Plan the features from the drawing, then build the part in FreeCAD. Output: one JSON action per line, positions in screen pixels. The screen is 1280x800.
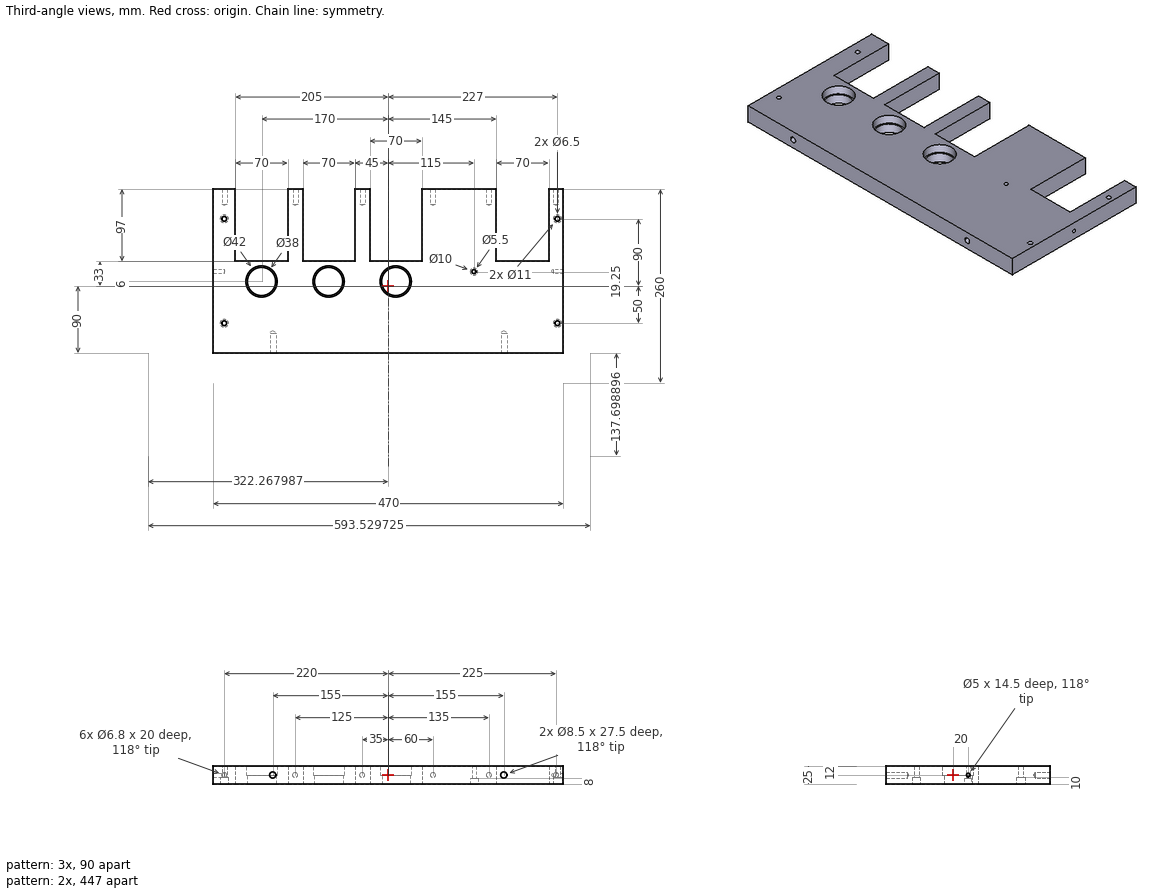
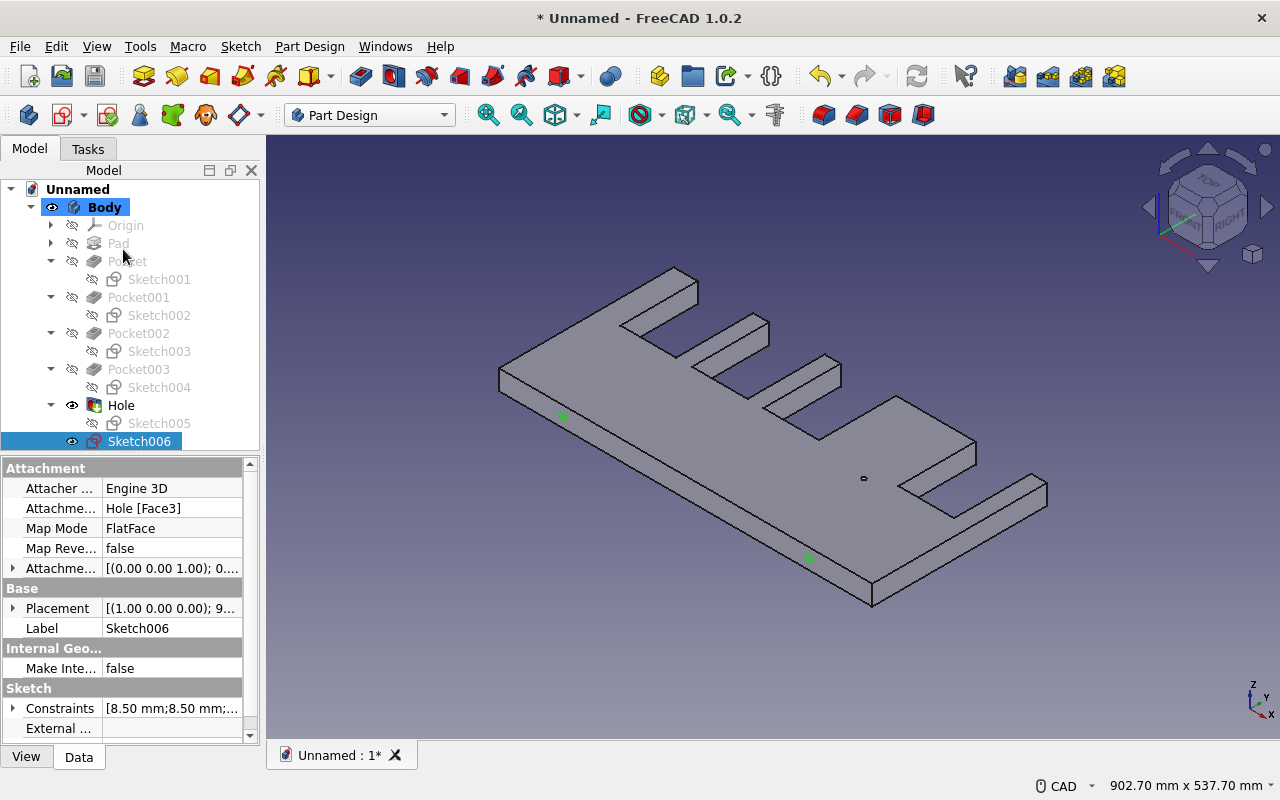
{"action": "left_click", "coordinate": [394, 76]}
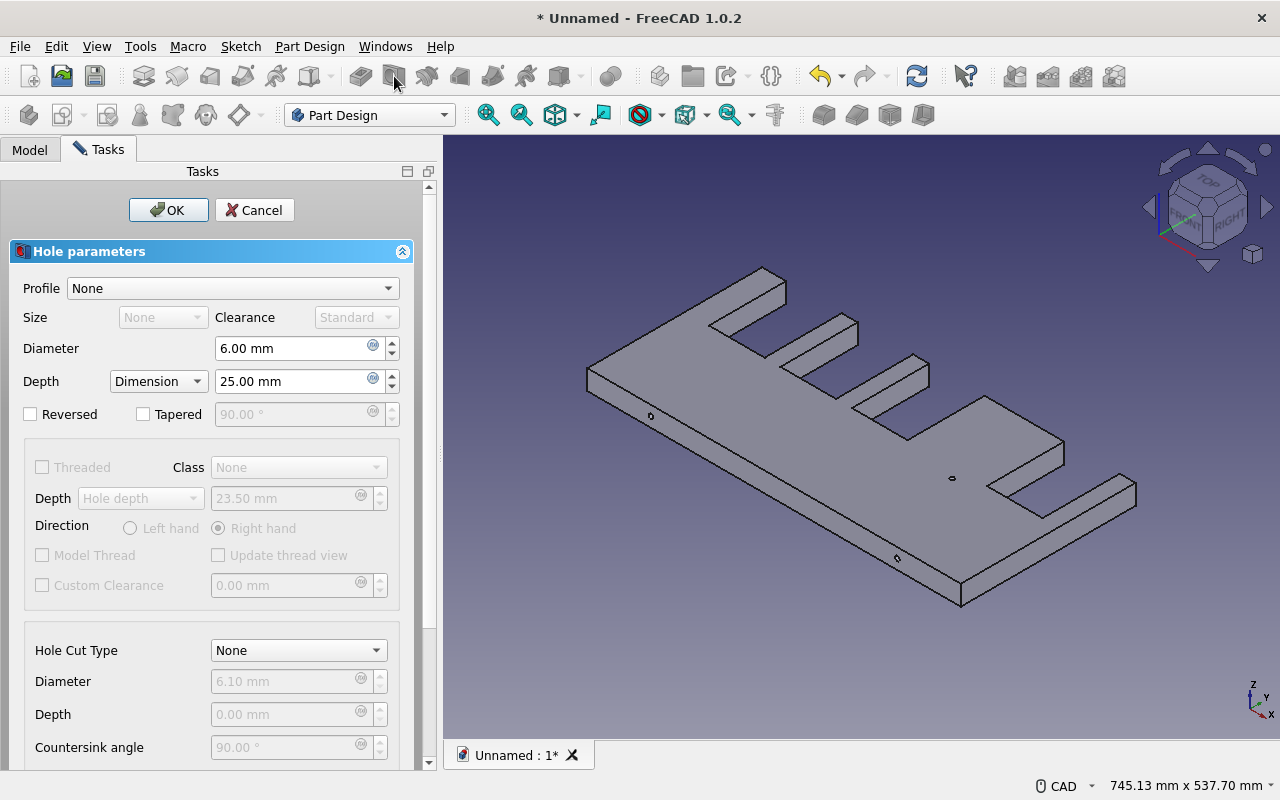
{"action": "triple_click", "coordinate": [300, 348]}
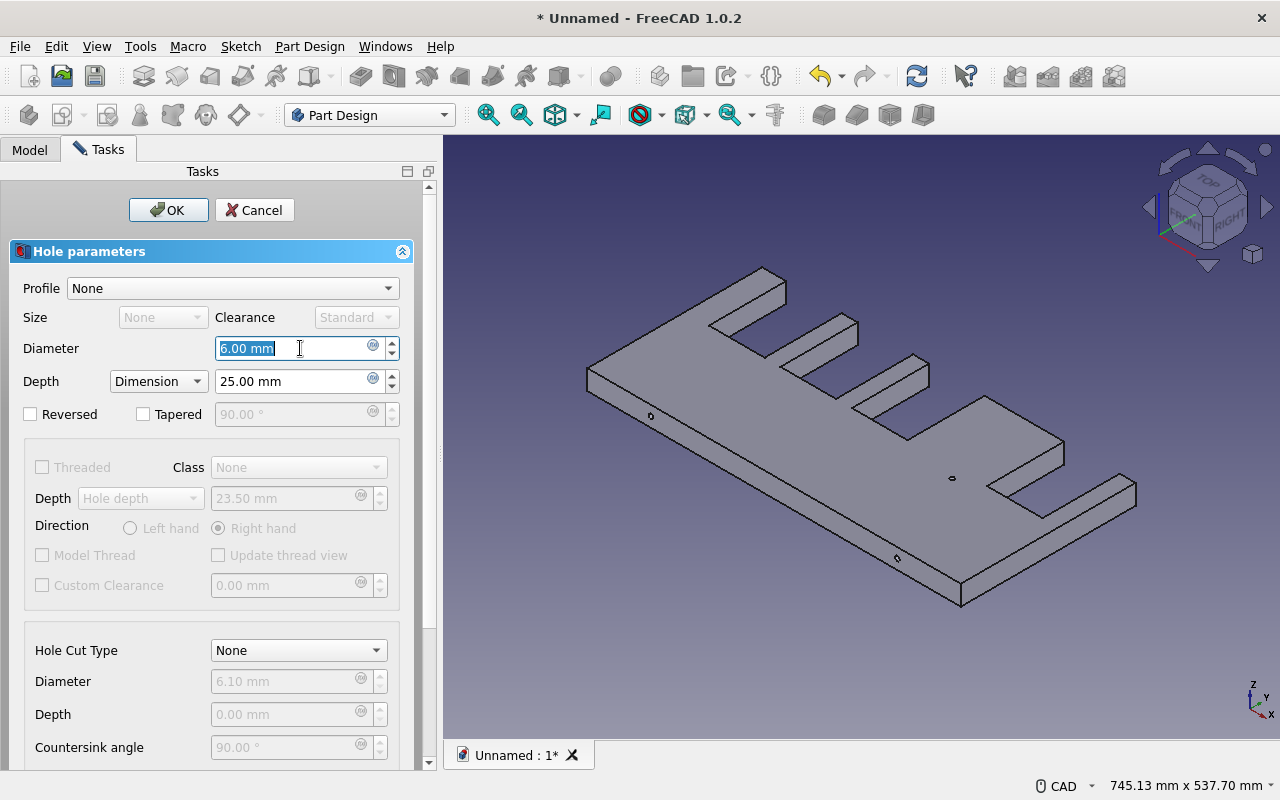
{"action": "type", "text": "8.5"}
{"action": "key", "text": "Tab"}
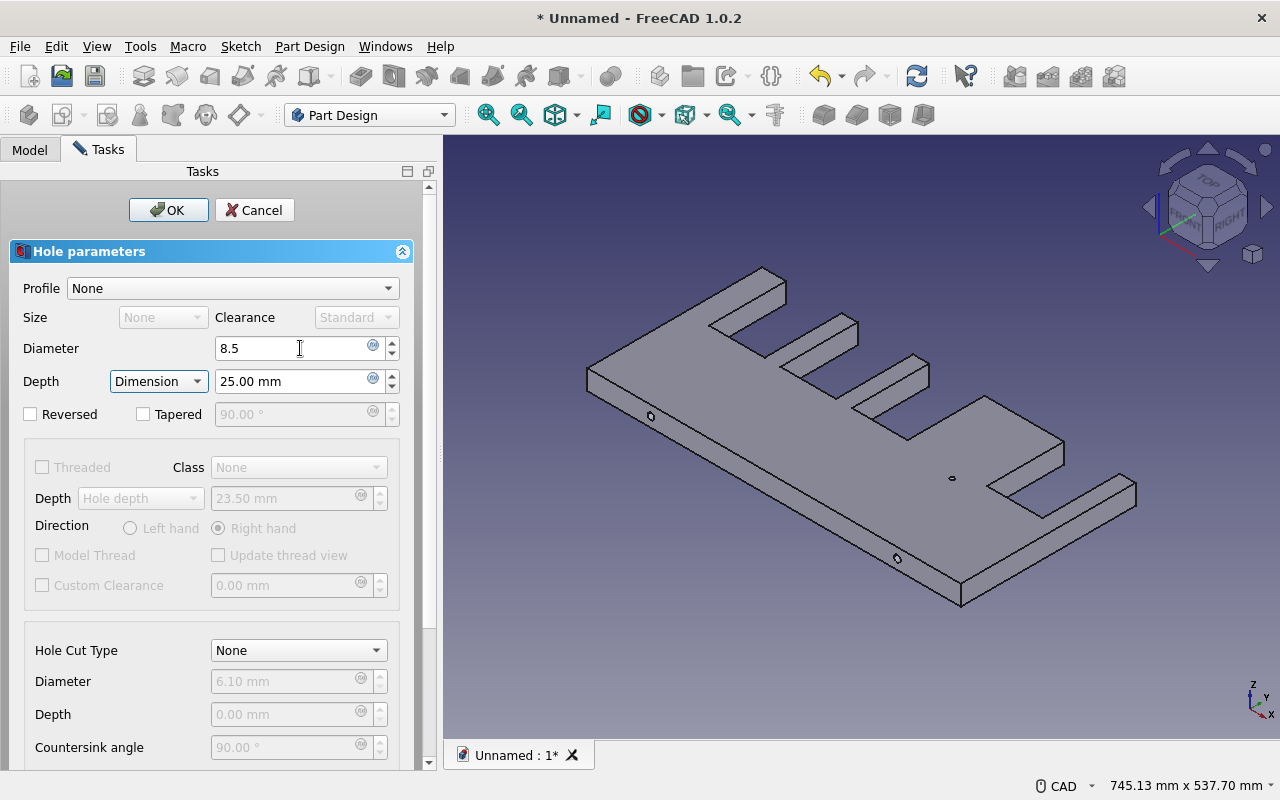
{"action": "triple_click", "coordinate": [300, 382]}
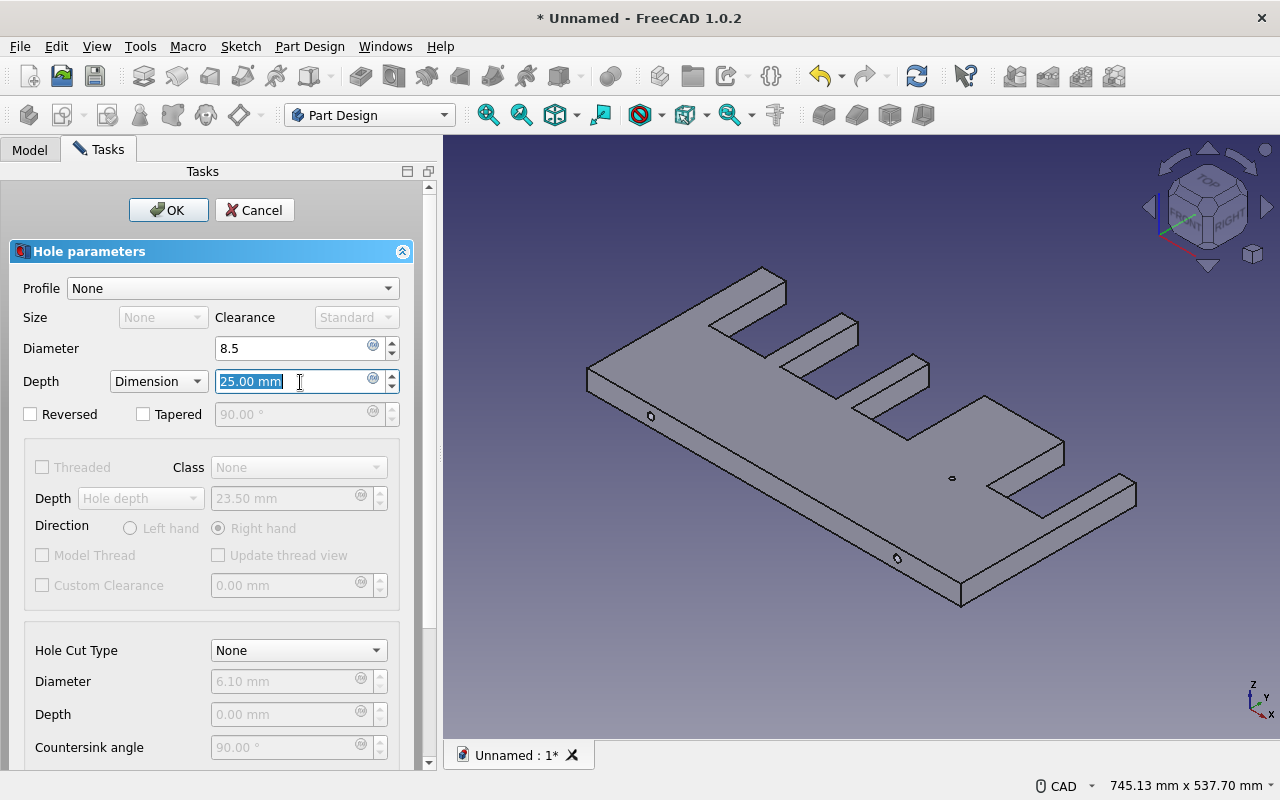
{"action": "type", "text": "27.5"}
{"action": "key", "text": "Tab"}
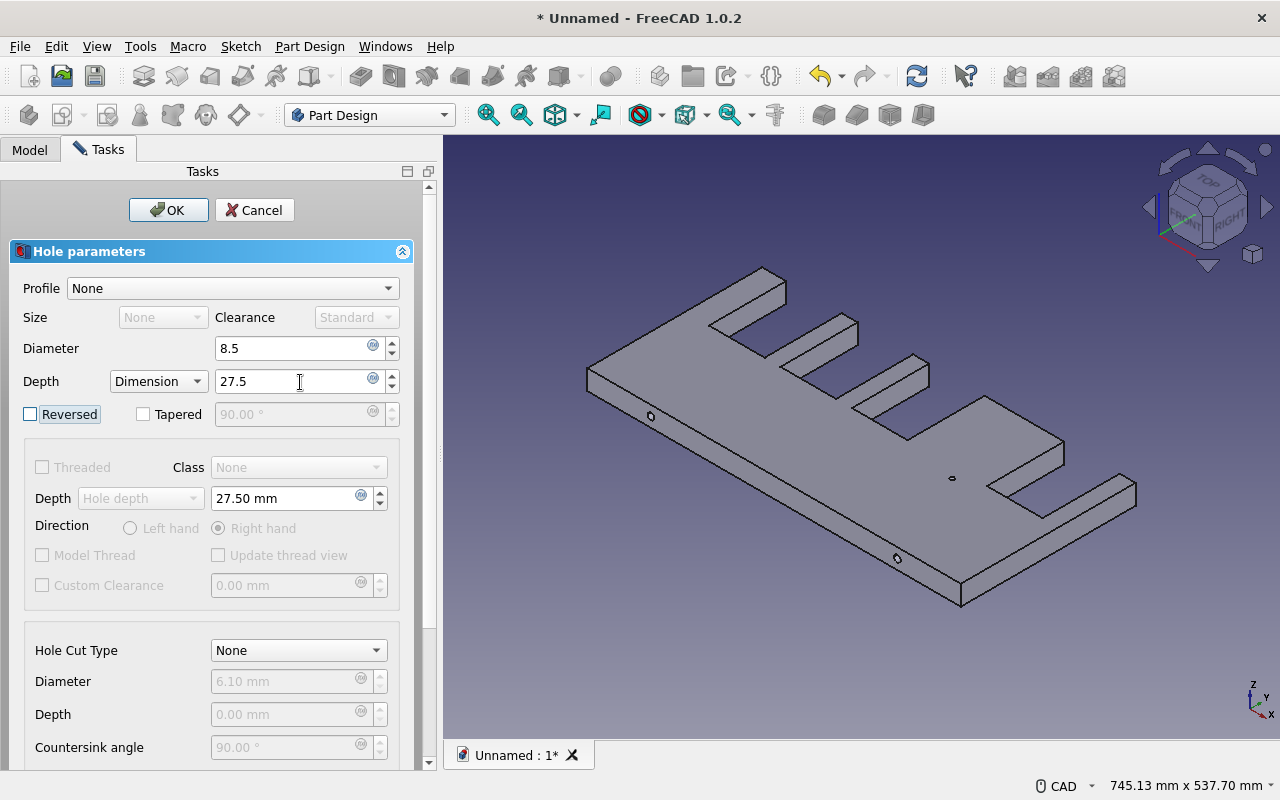
{"action": "left_click", "coordinate": [169, 210]}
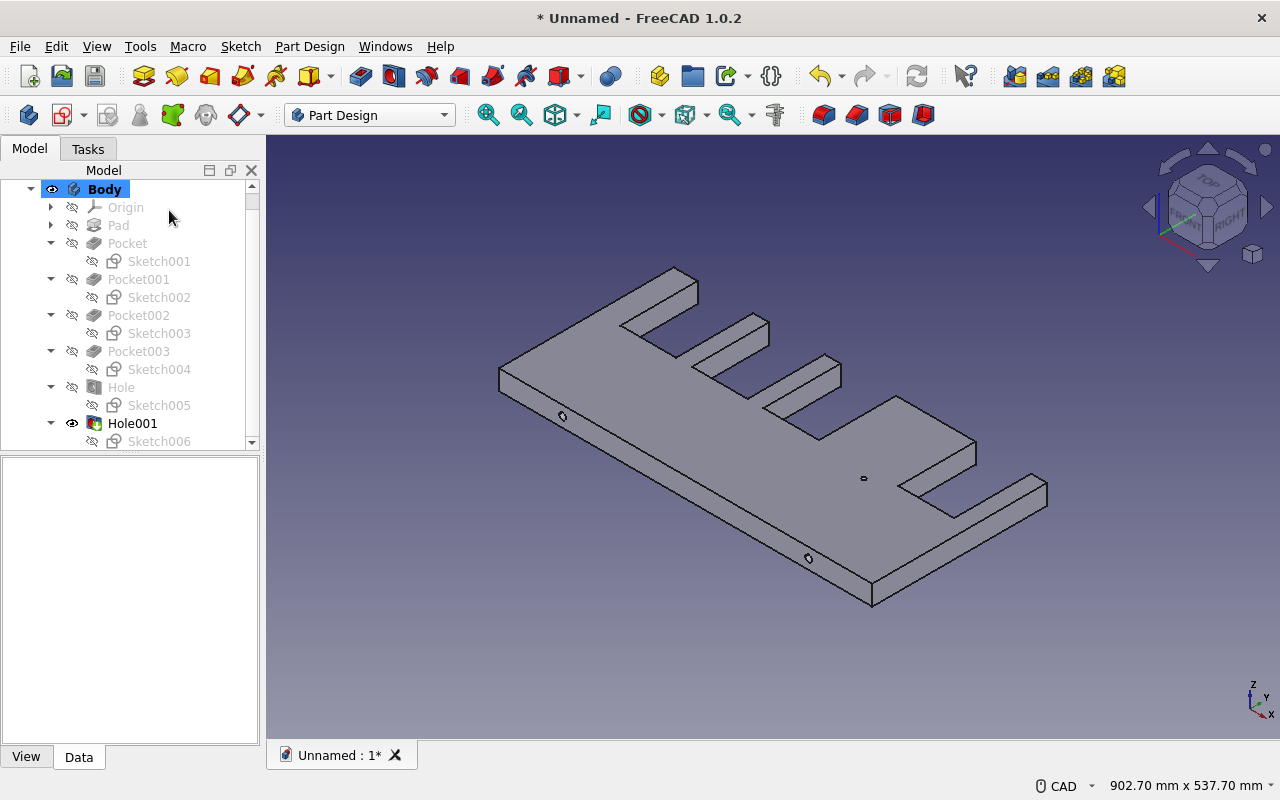
{"action": "left_click", "coordinate": [801, 470]}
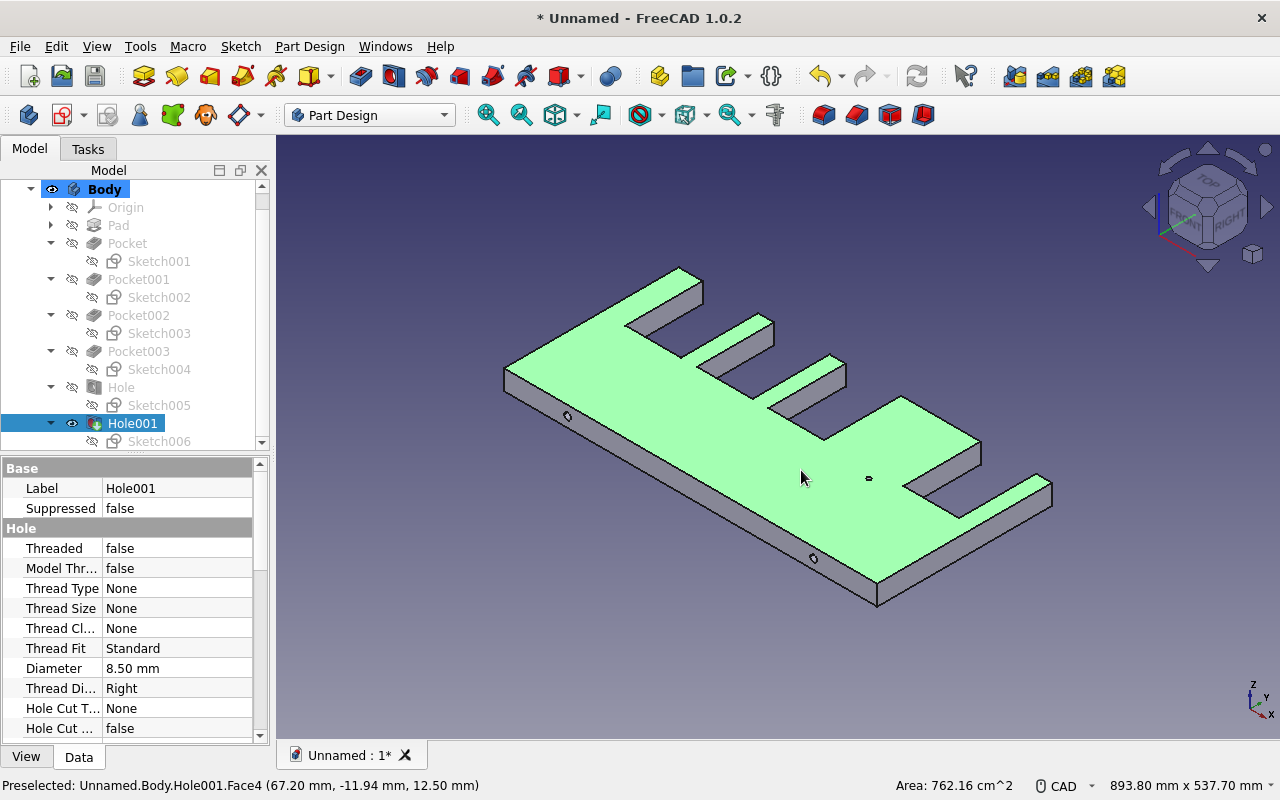
{"action": "left_click", "coordinate": [62, 116]}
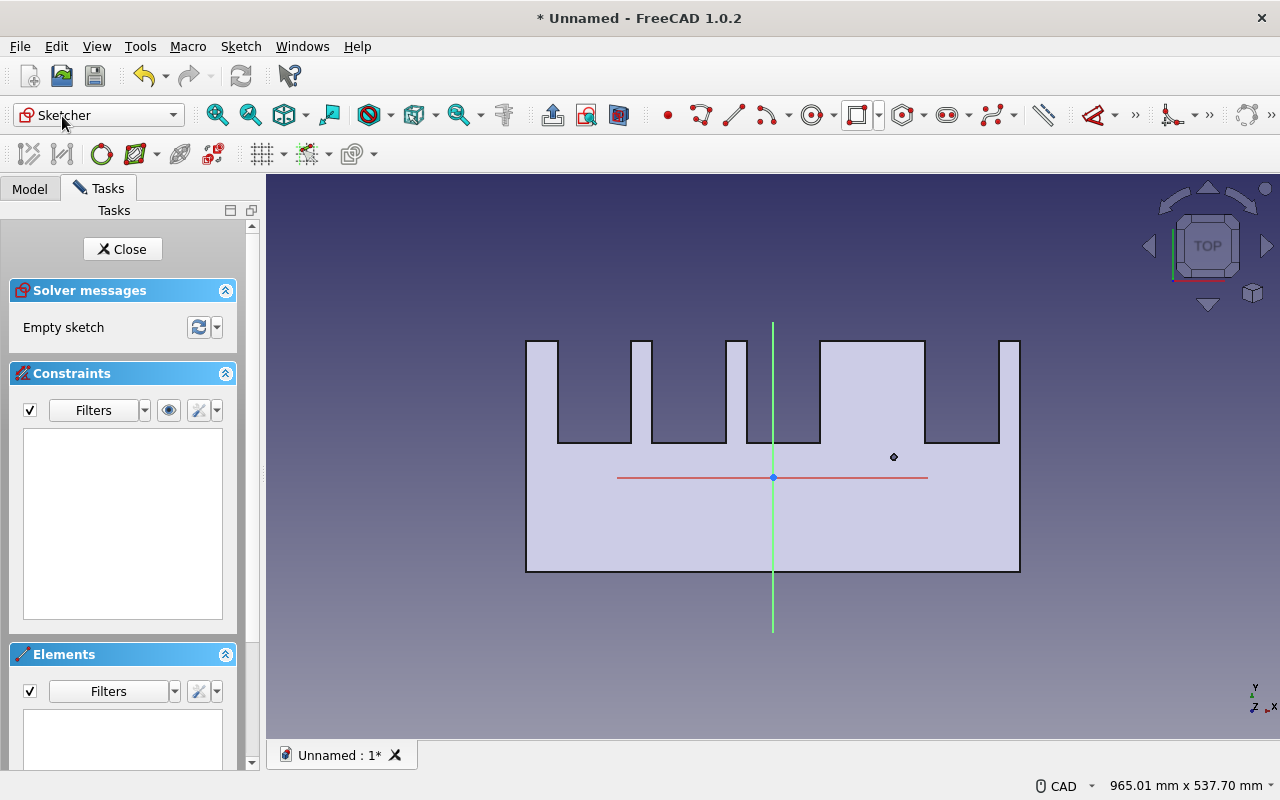
{"action": "scroll", "coordinate": [581, 473], "scroll_direction": "up", "scroll_amount": 11}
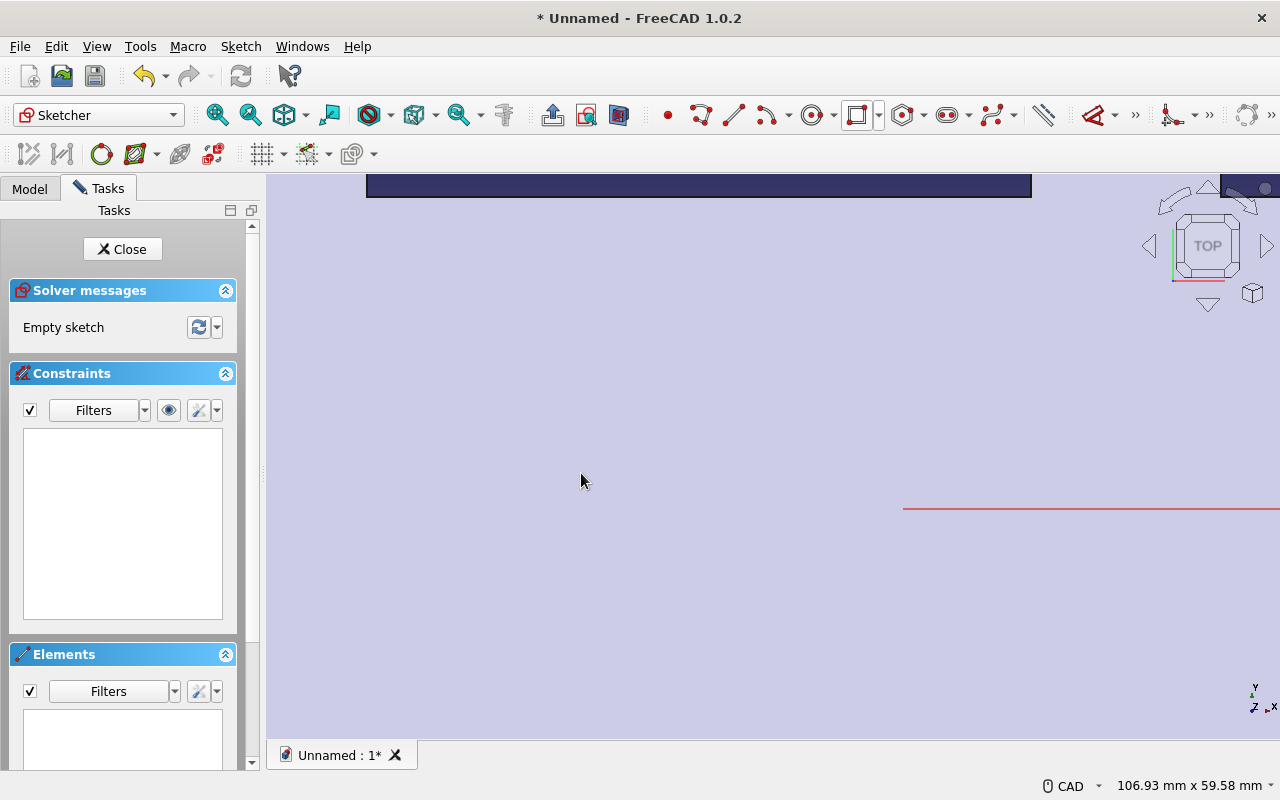
{"action": "left_click", "coordinate": [812, 116]}